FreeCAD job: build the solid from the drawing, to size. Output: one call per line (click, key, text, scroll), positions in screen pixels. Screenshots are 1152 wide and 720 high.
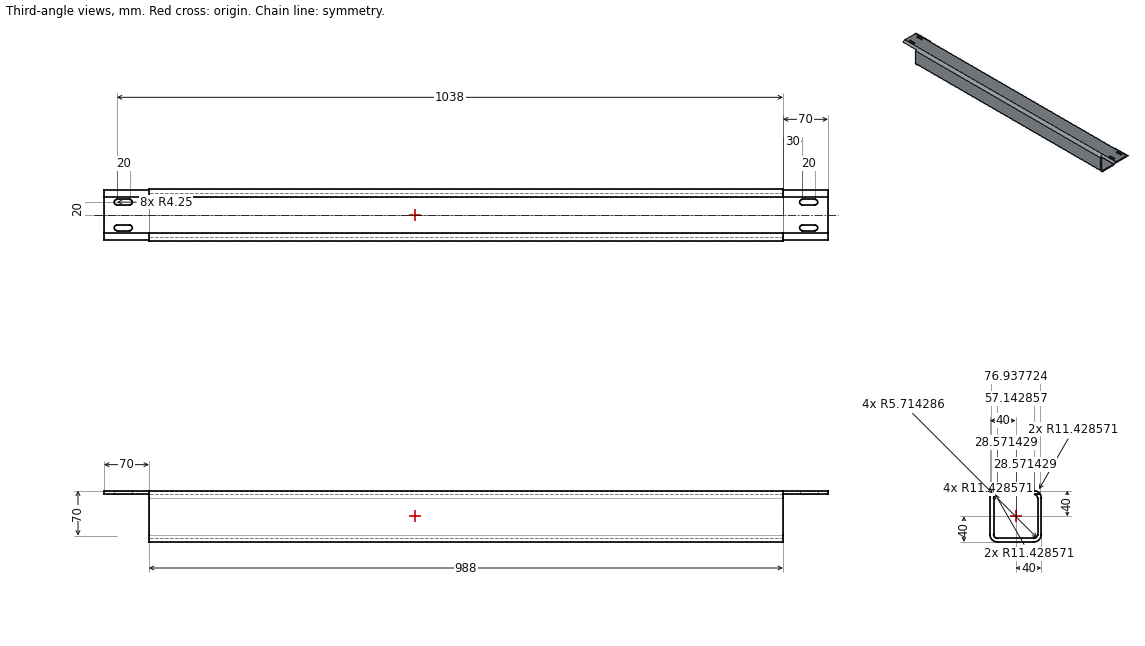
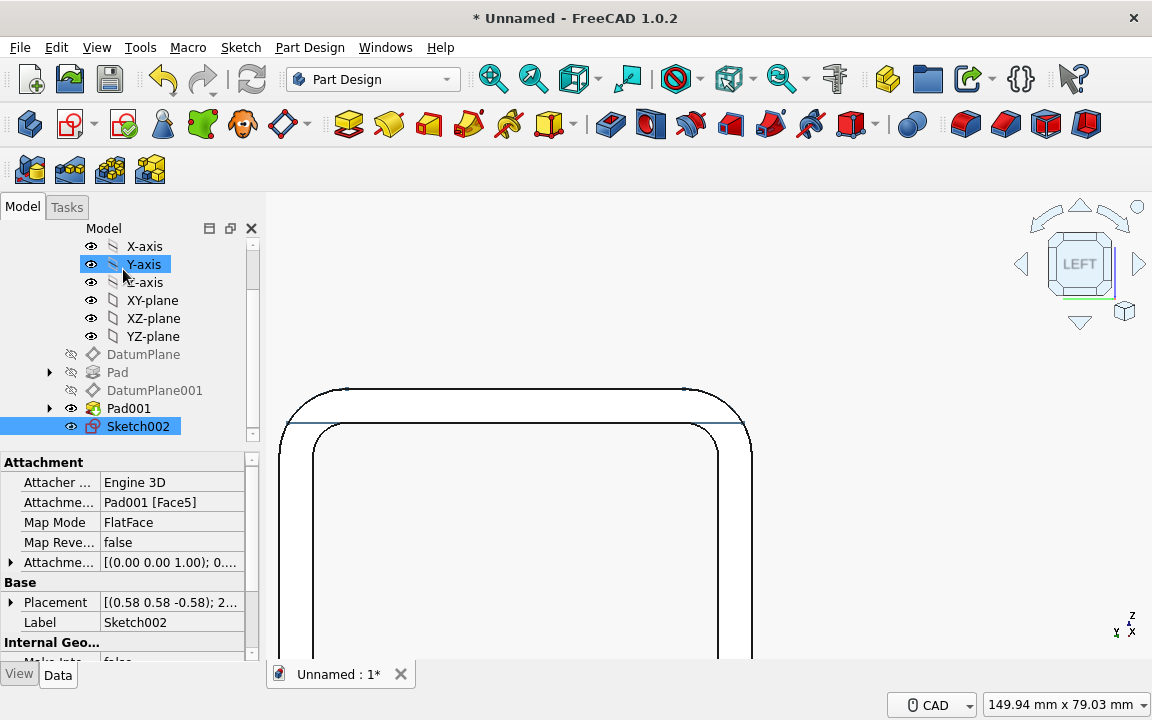
click(350, 124)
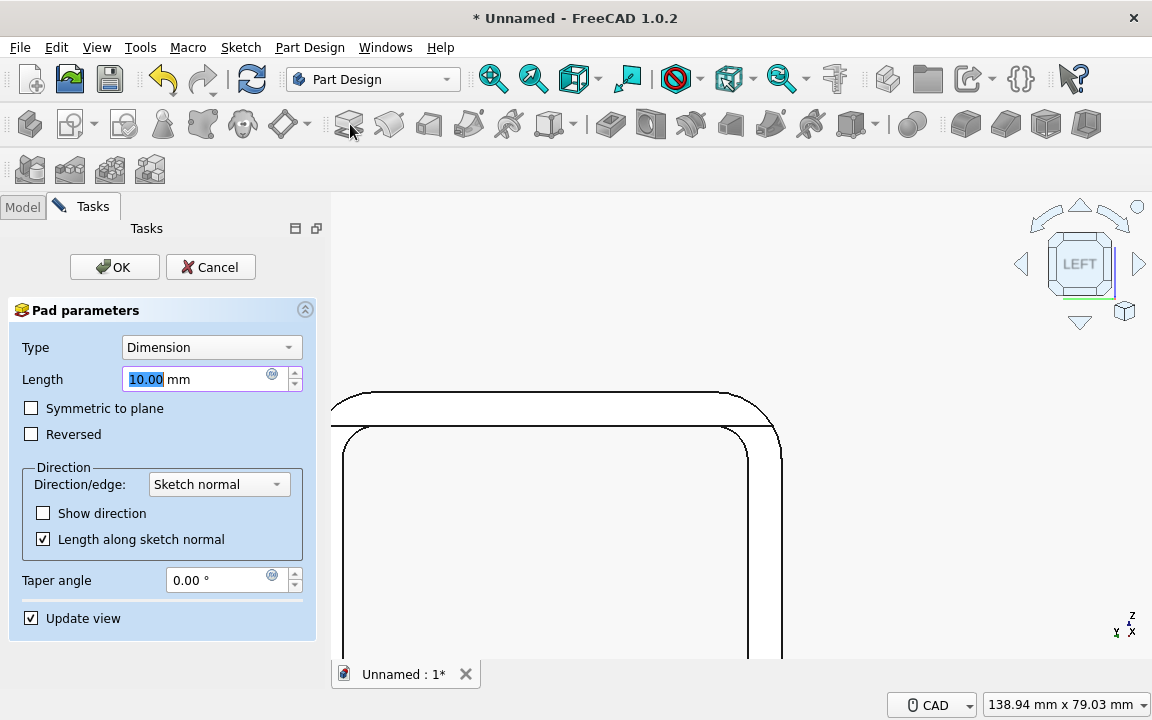
text(70)
key(Tab)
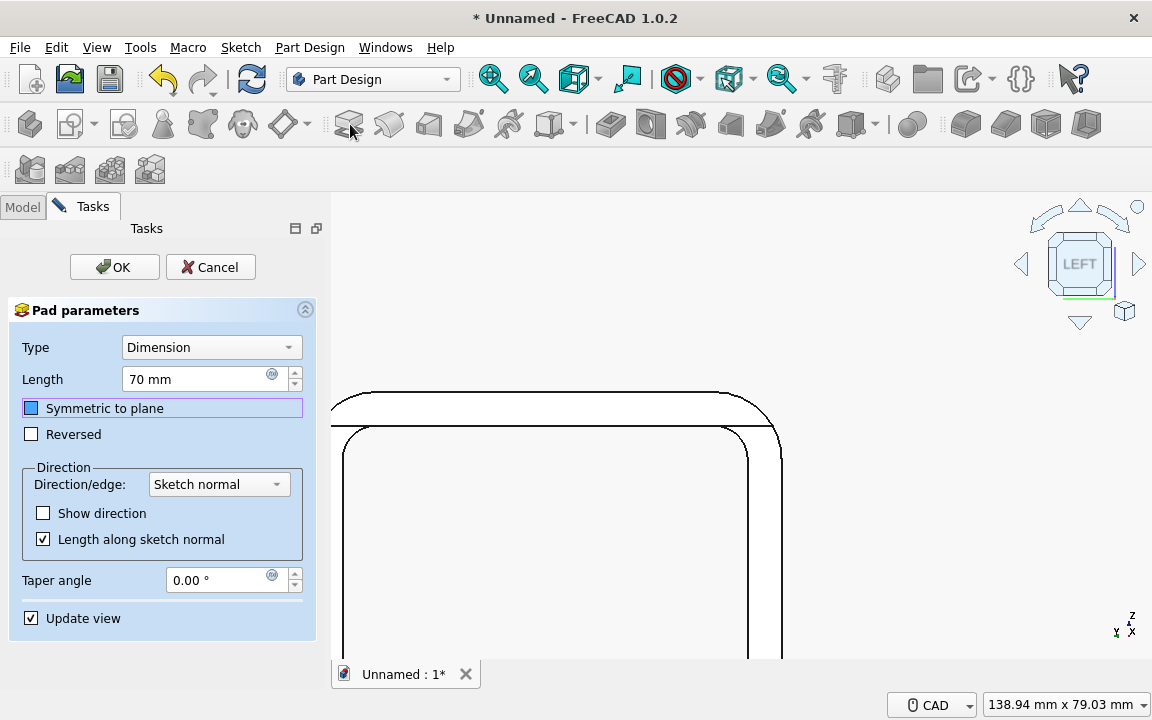
click(115, 267)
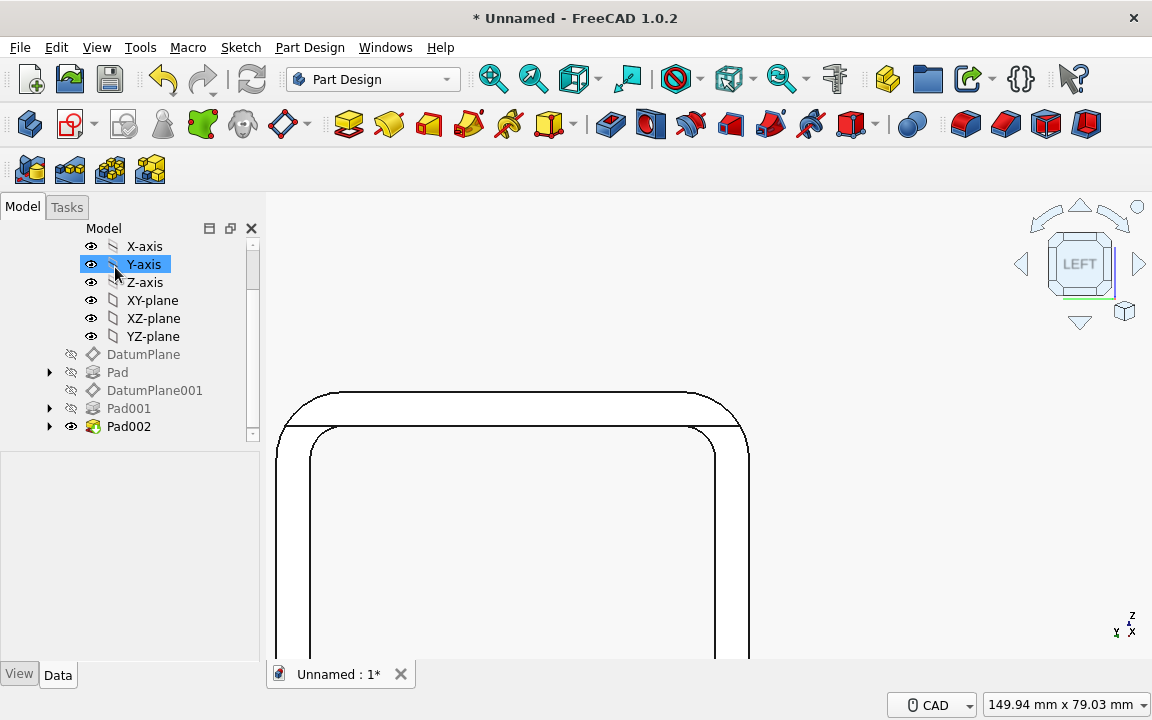
key(v)
key(f)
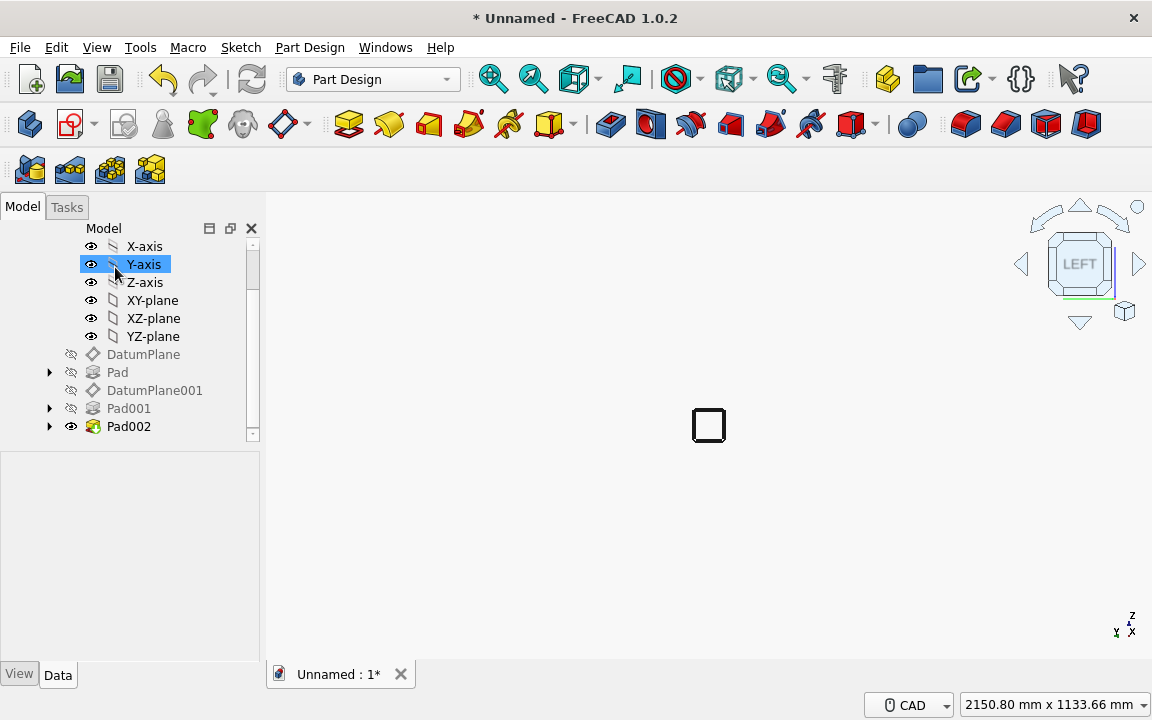
key(0)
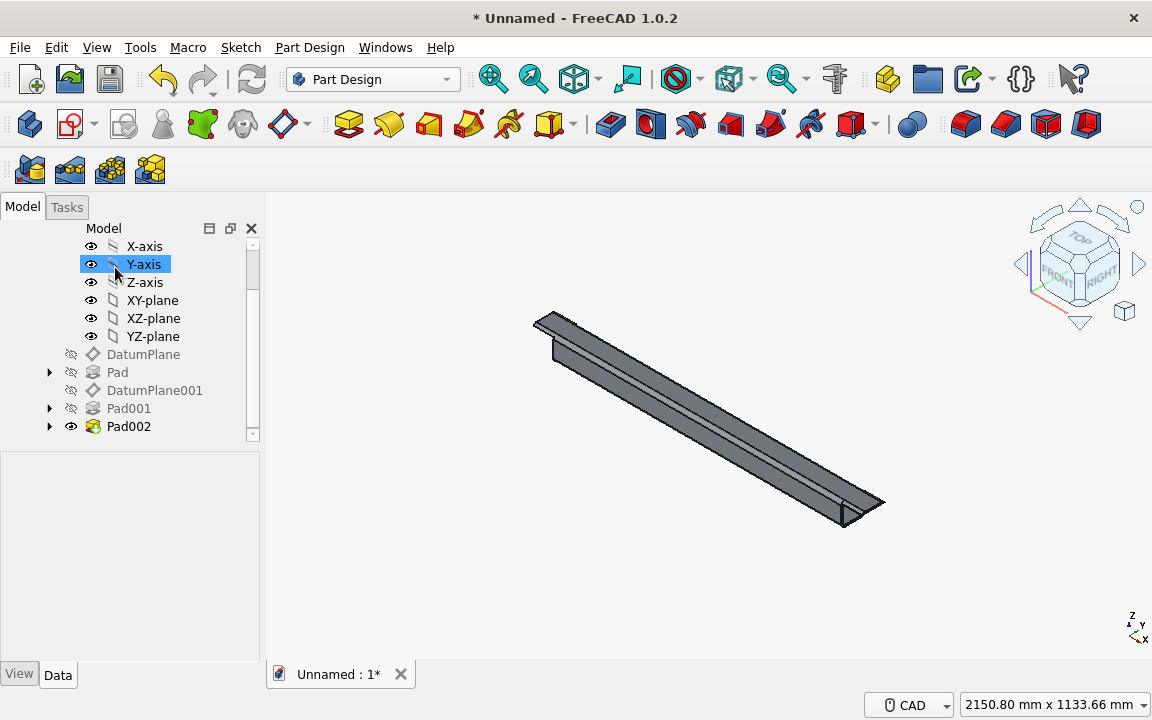
key(2)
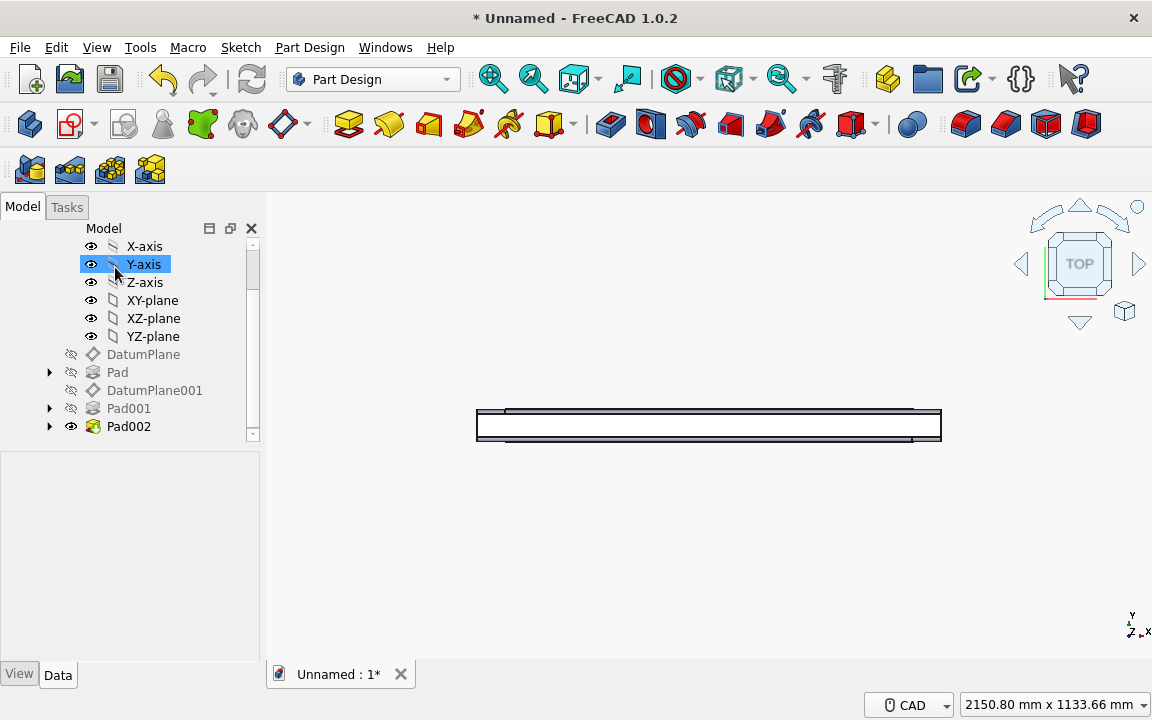
click(908, 424)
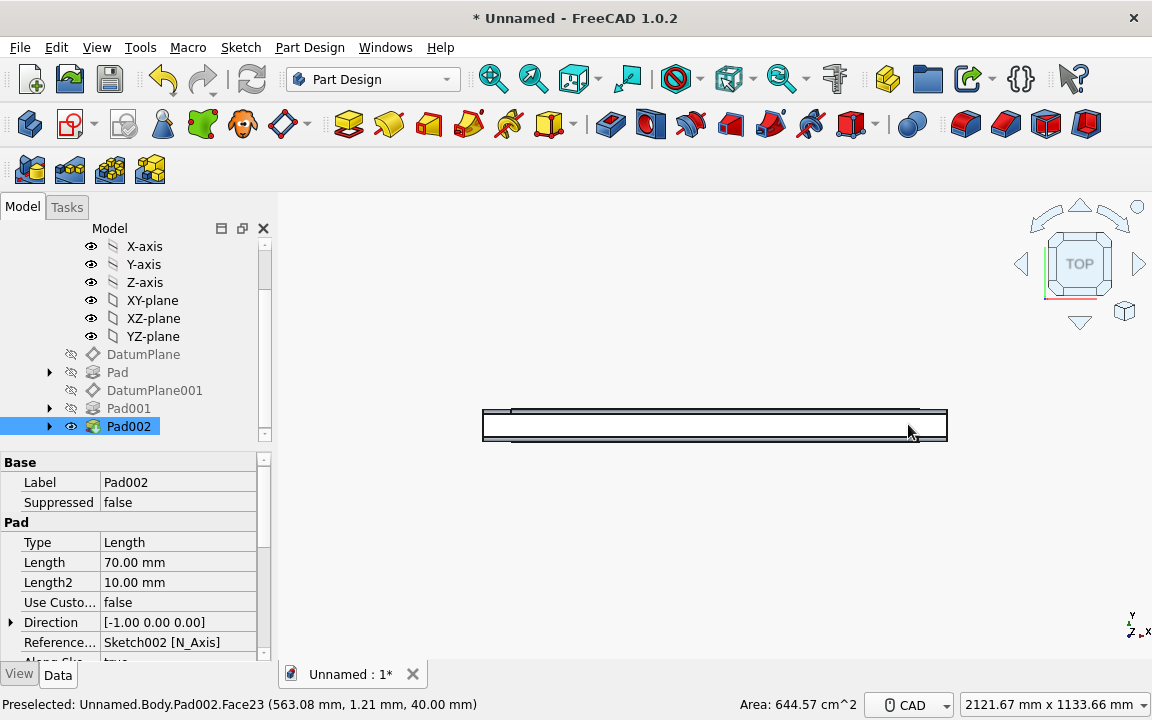
click(70, 124)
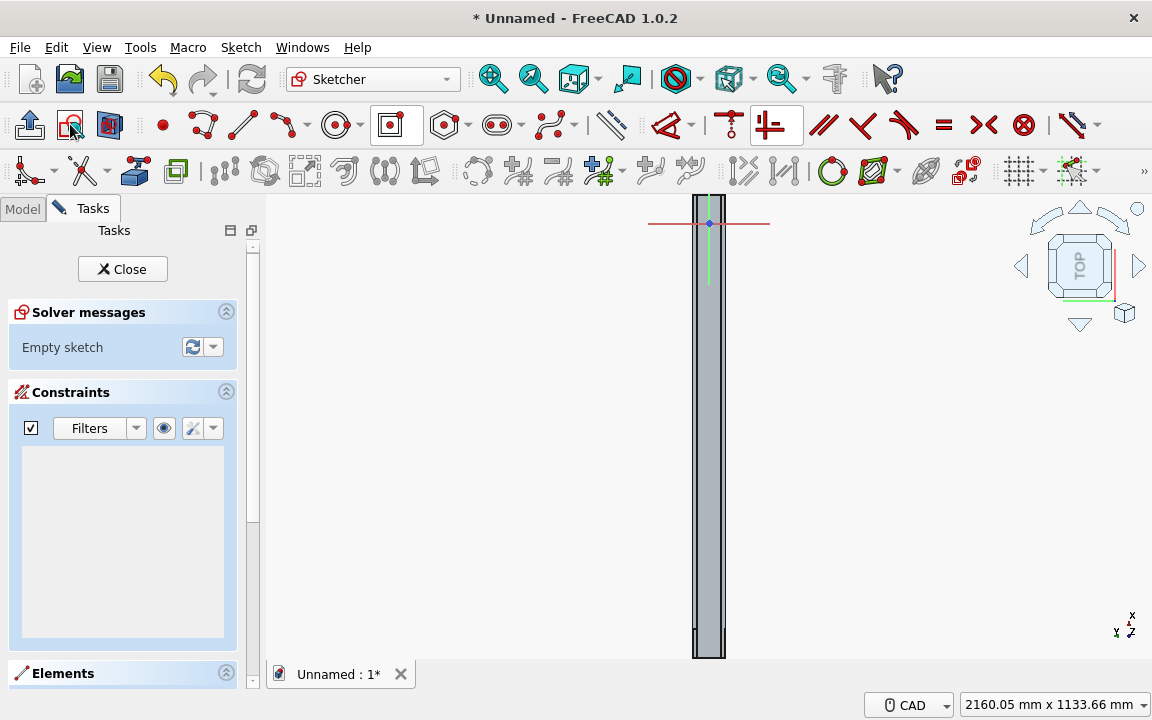
scroll(501, 427, down, 2)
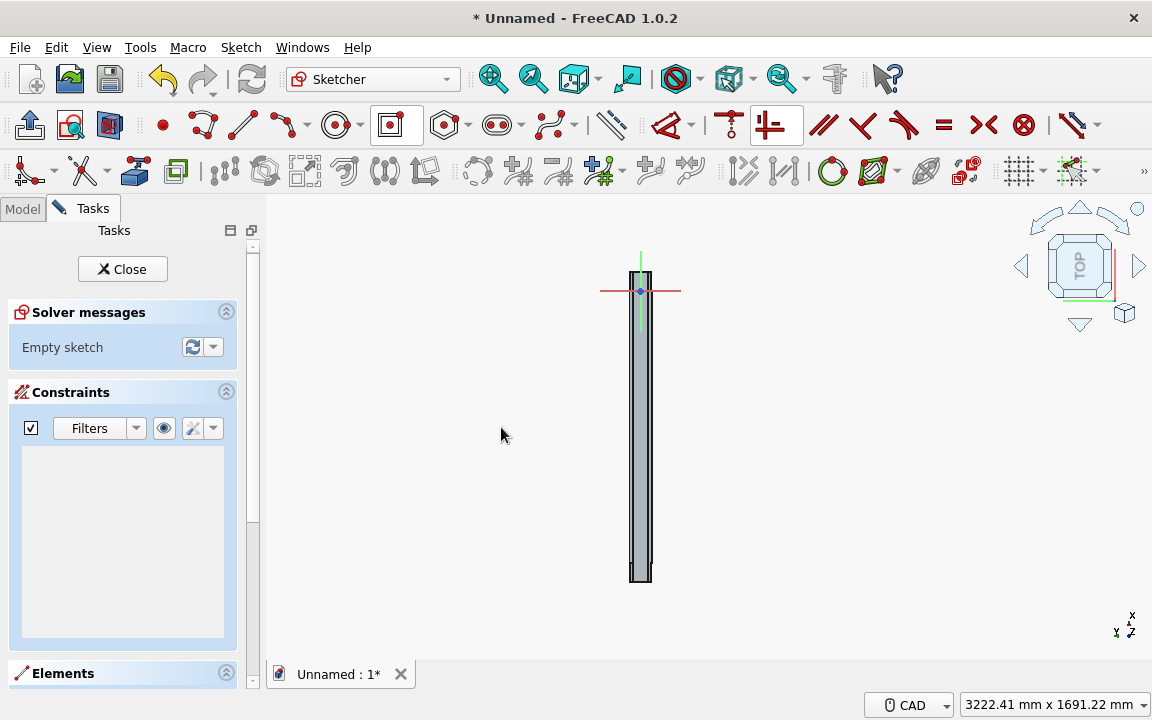
click(498, 126)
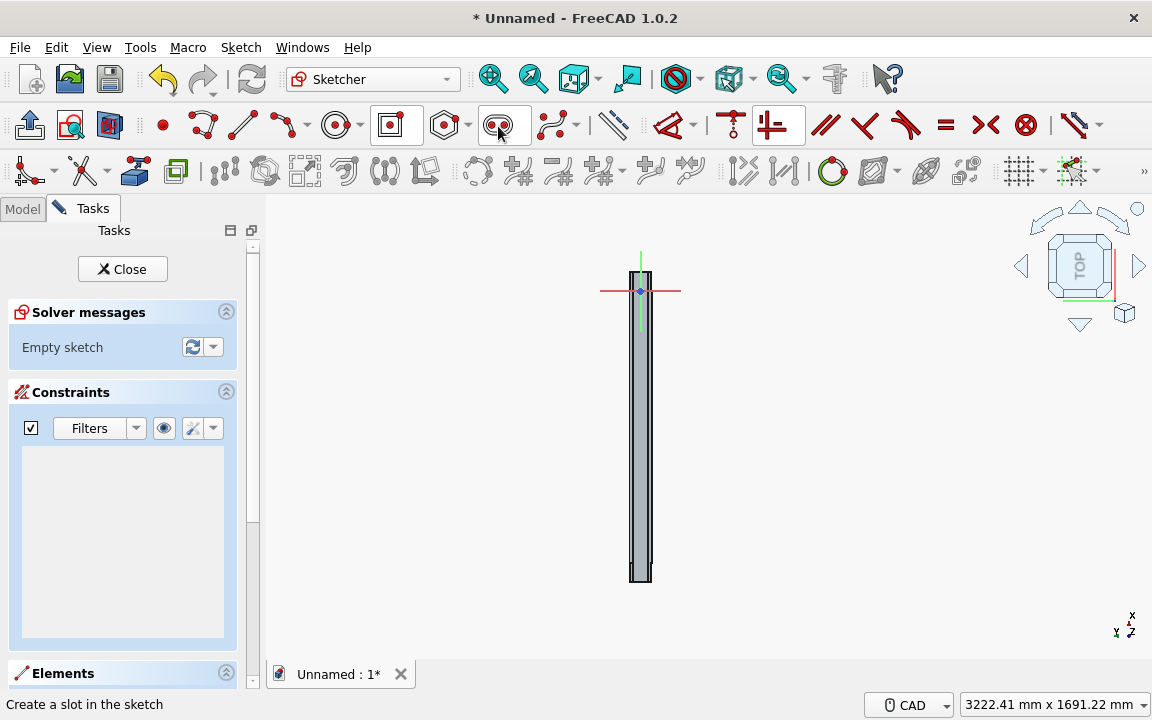
scroll(635, 576, up, 15)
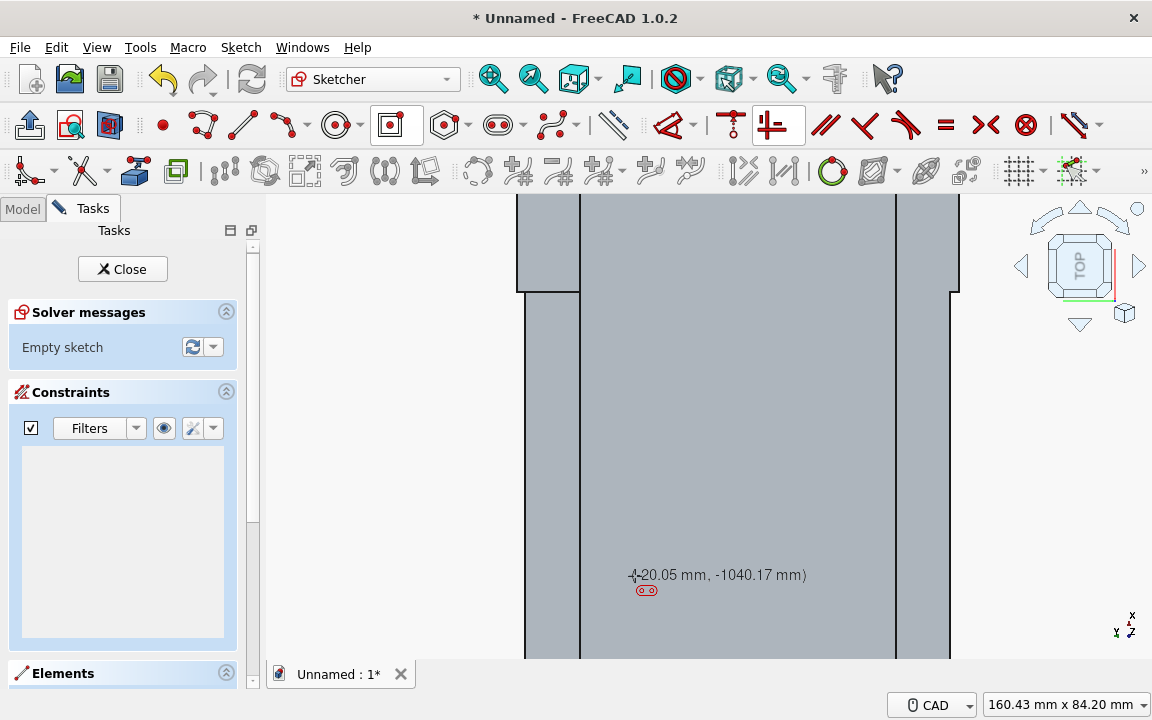
scroll(635, 576, down, 15)